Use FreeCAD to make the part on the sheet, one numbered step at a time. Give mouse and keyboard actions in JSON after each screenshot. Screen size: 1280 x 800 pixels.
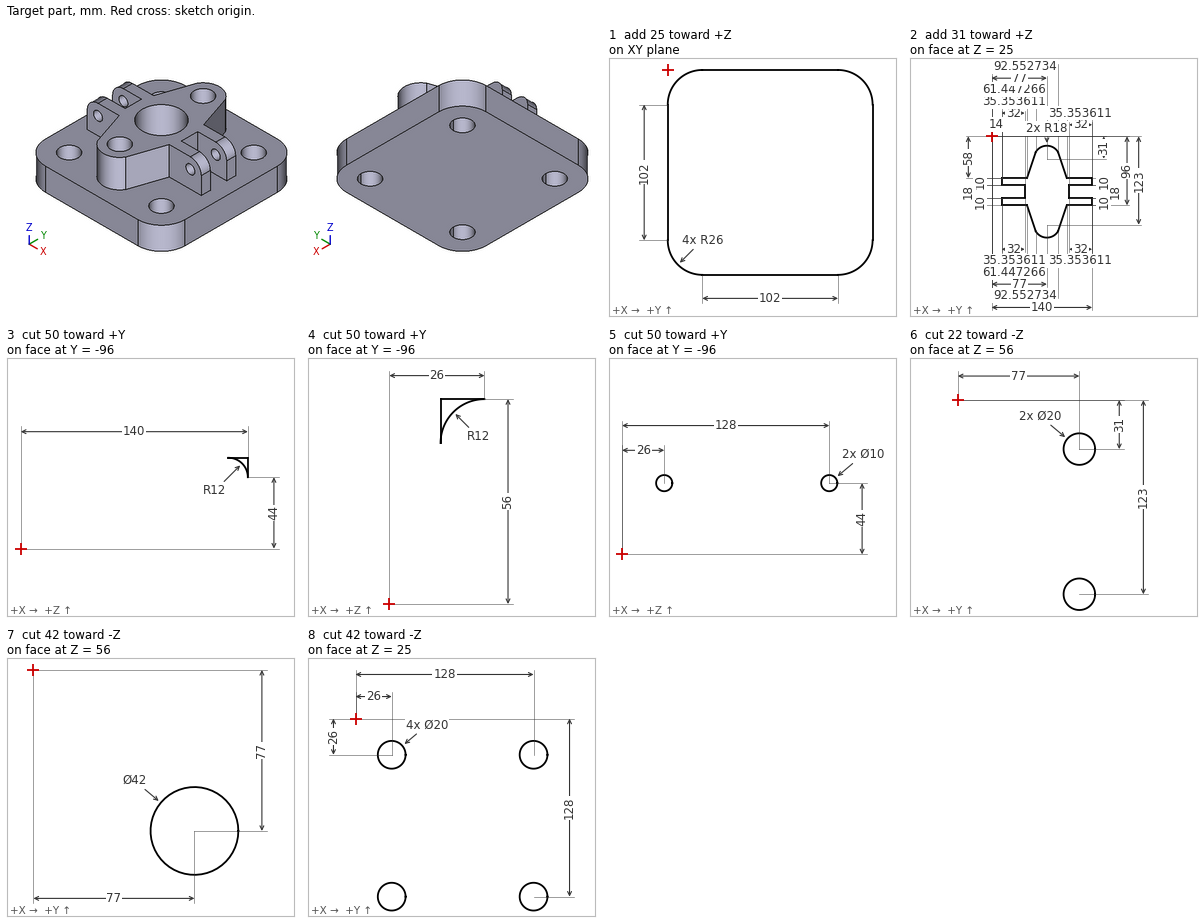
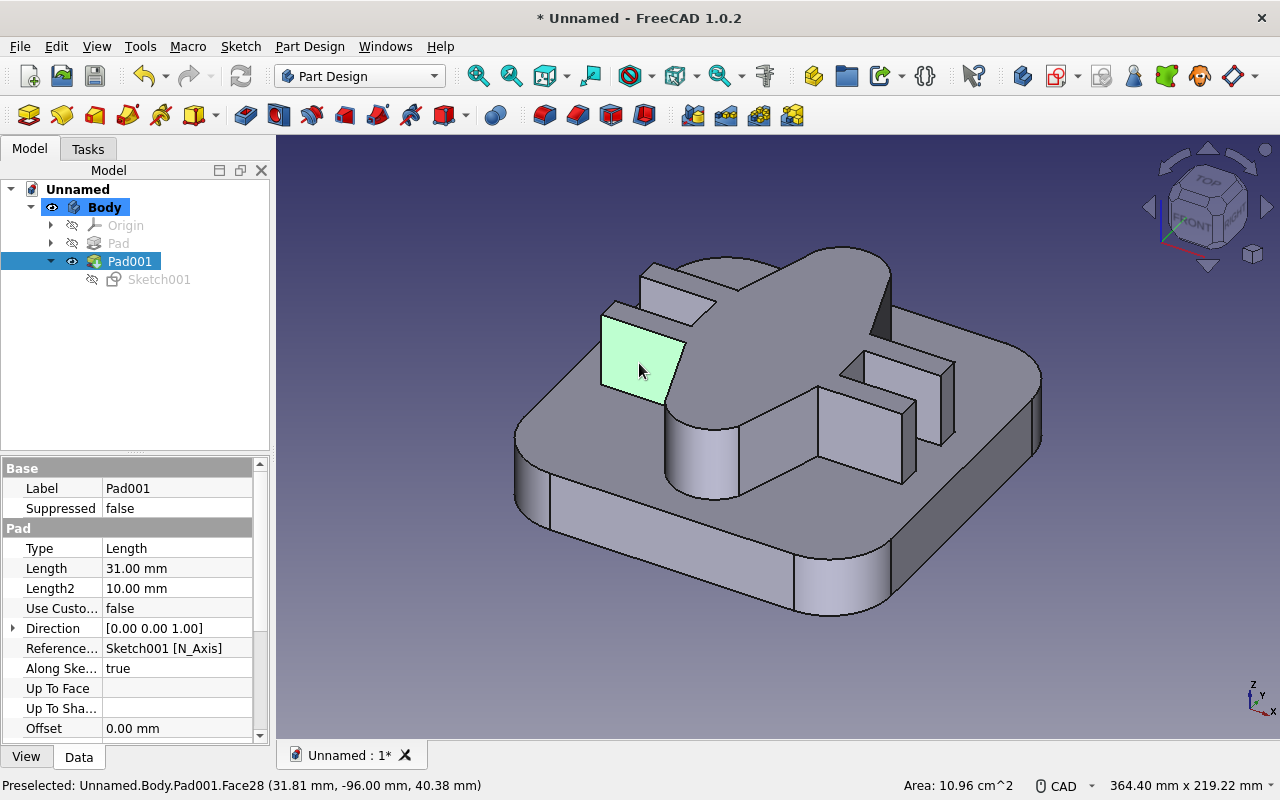
{"action": "left_click", "coordinate": [1056, 76]}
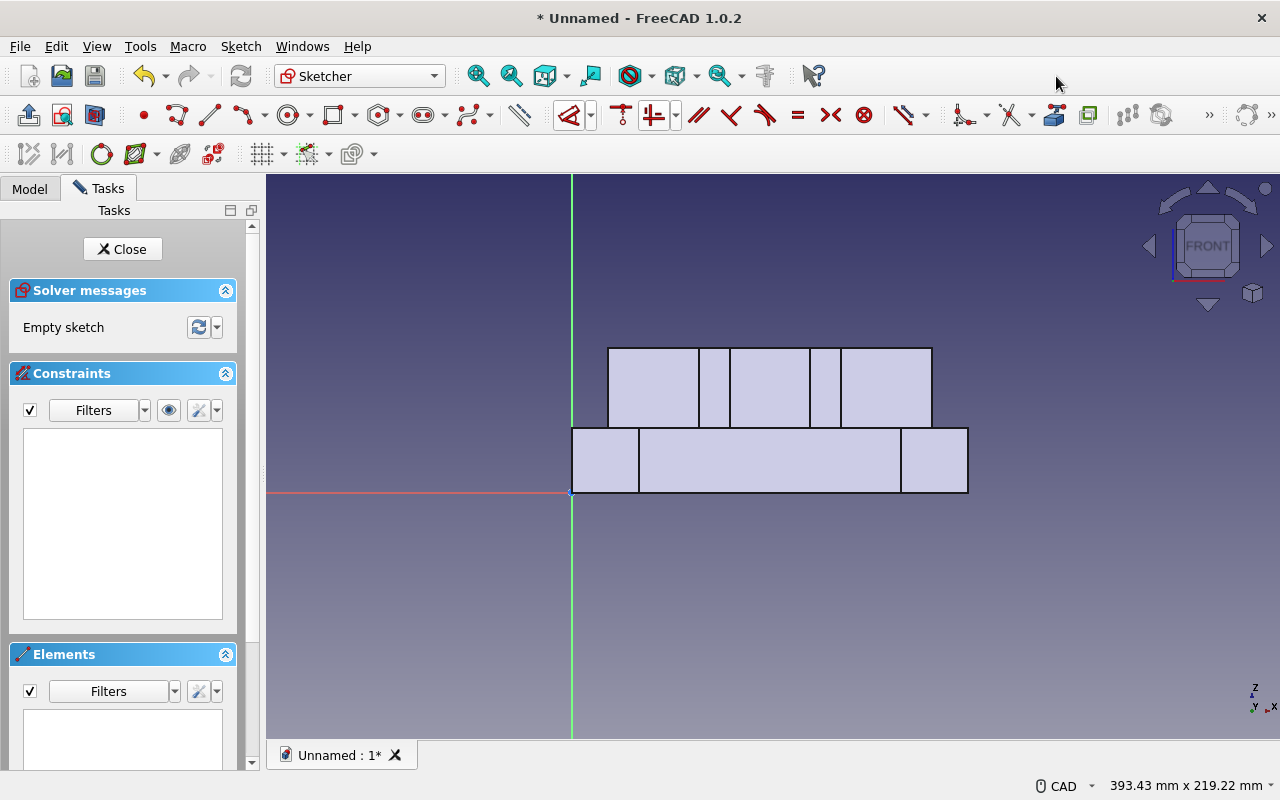
{"action": "scroll", "coordinate": [938, 354], "scroll_direction": "up", "scroll_amount": 12}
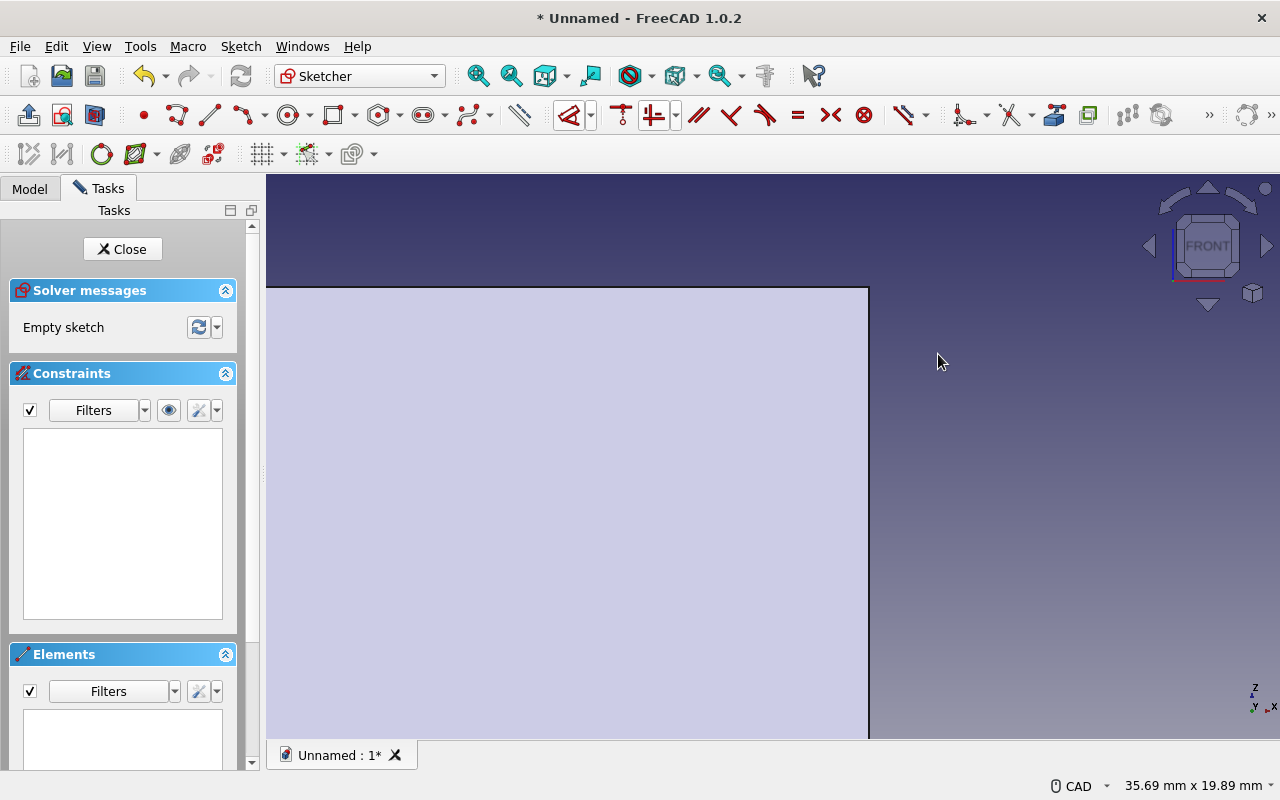
{"action": "left_click", "coordinate": [177, 116]}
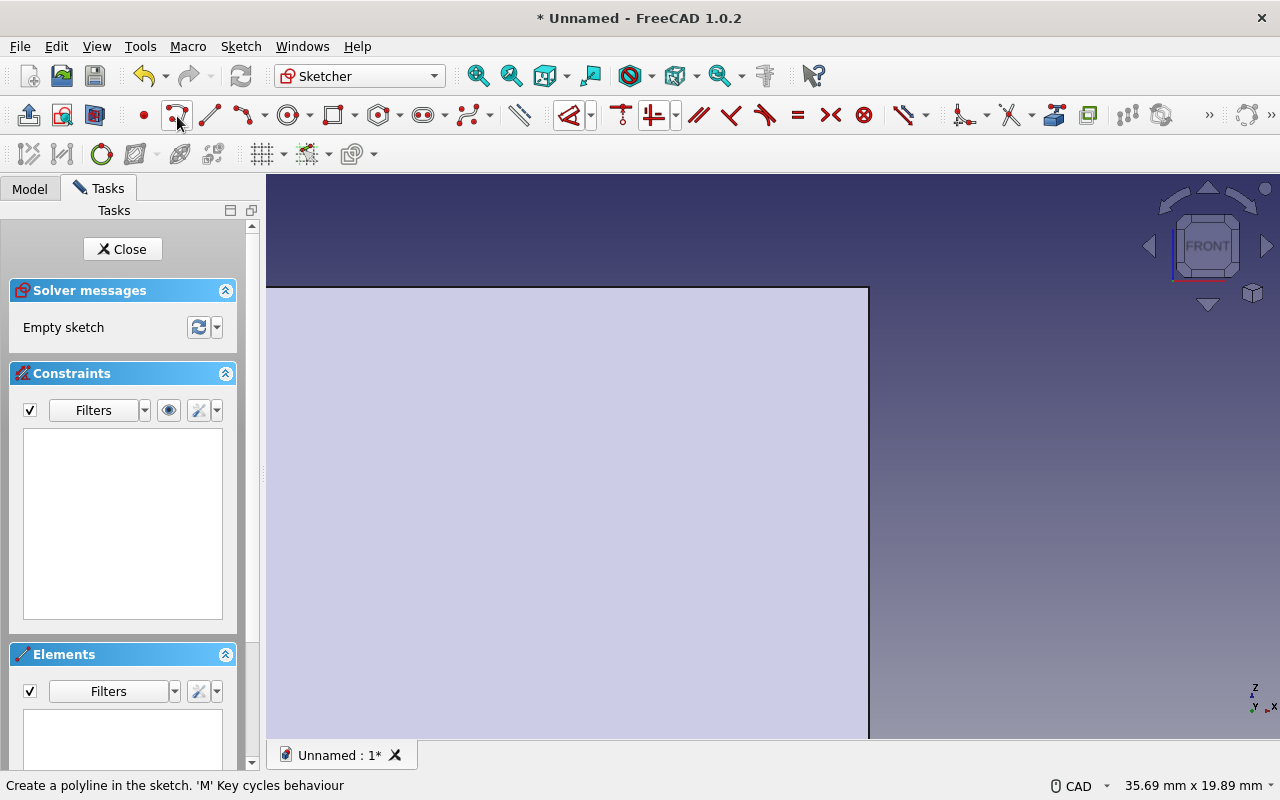
{"action": "left_click", "coordinate": [869, 628]}
{"action": "left_click", "coordinate": [869, 287]}
{"action": "left_click", "coordinate": [528, 287]}
{"action": "right_click", "coordinate": [528, 287]}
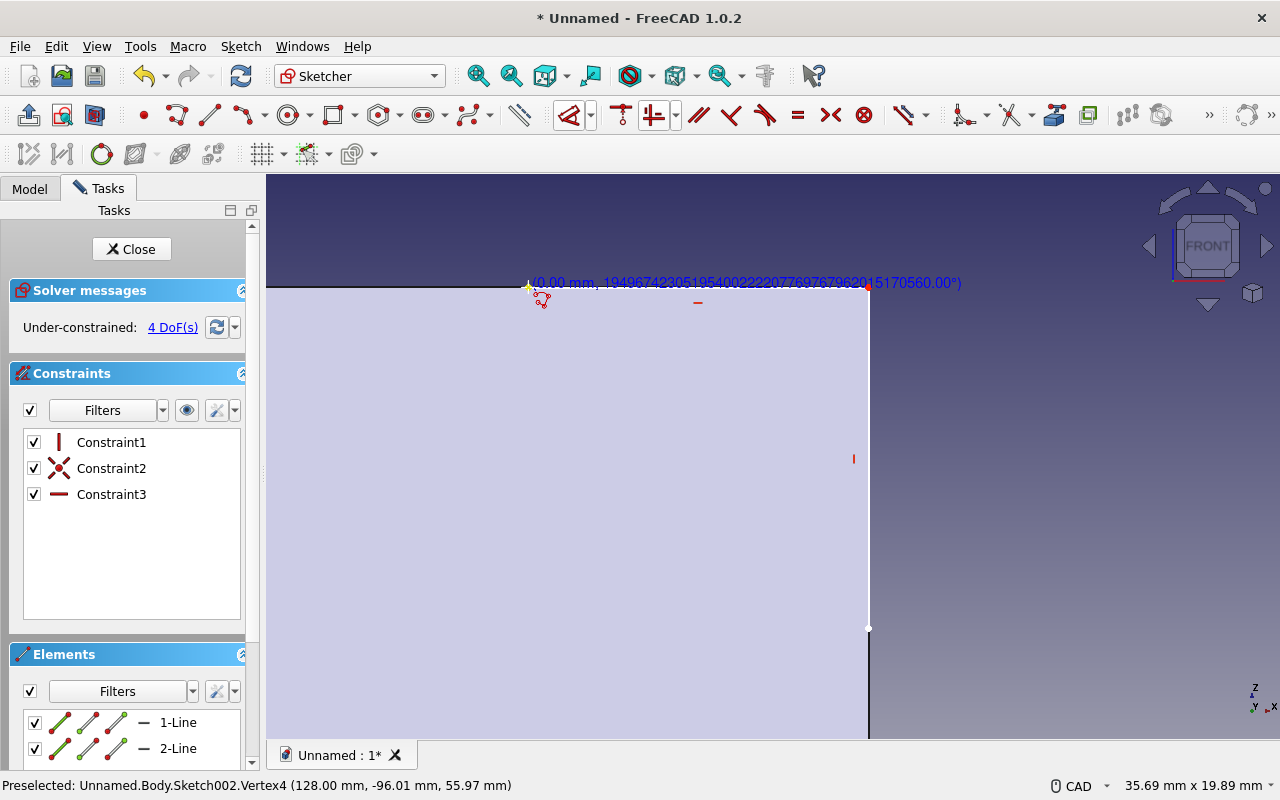
{"action": "left_click", "coordinate": [242, 116]}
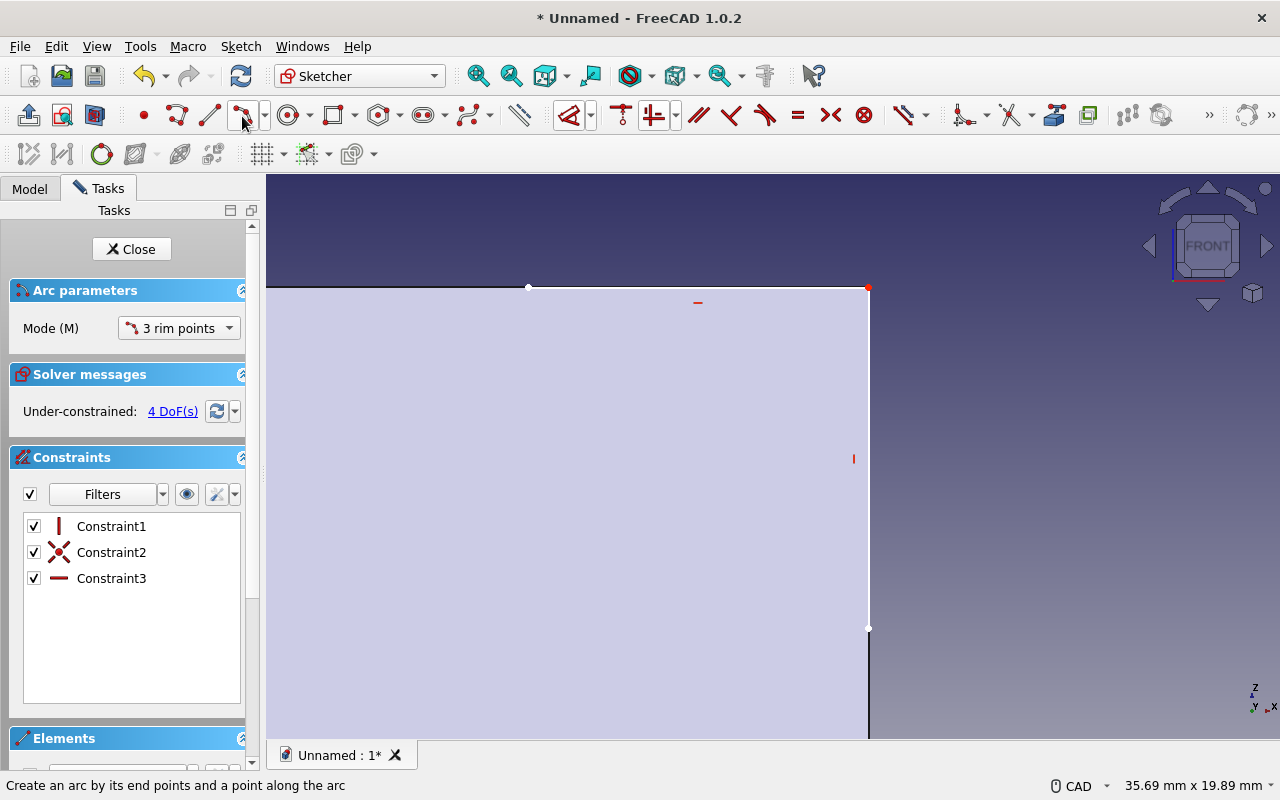
{"action": "left_click", "coordinate": [528, 288]}
{"action": "left_click", "coordinate": [869, 629]}
{"action": "left_click", "coordinate": [769, 387]}
{"action": "key", "text": "Escape"}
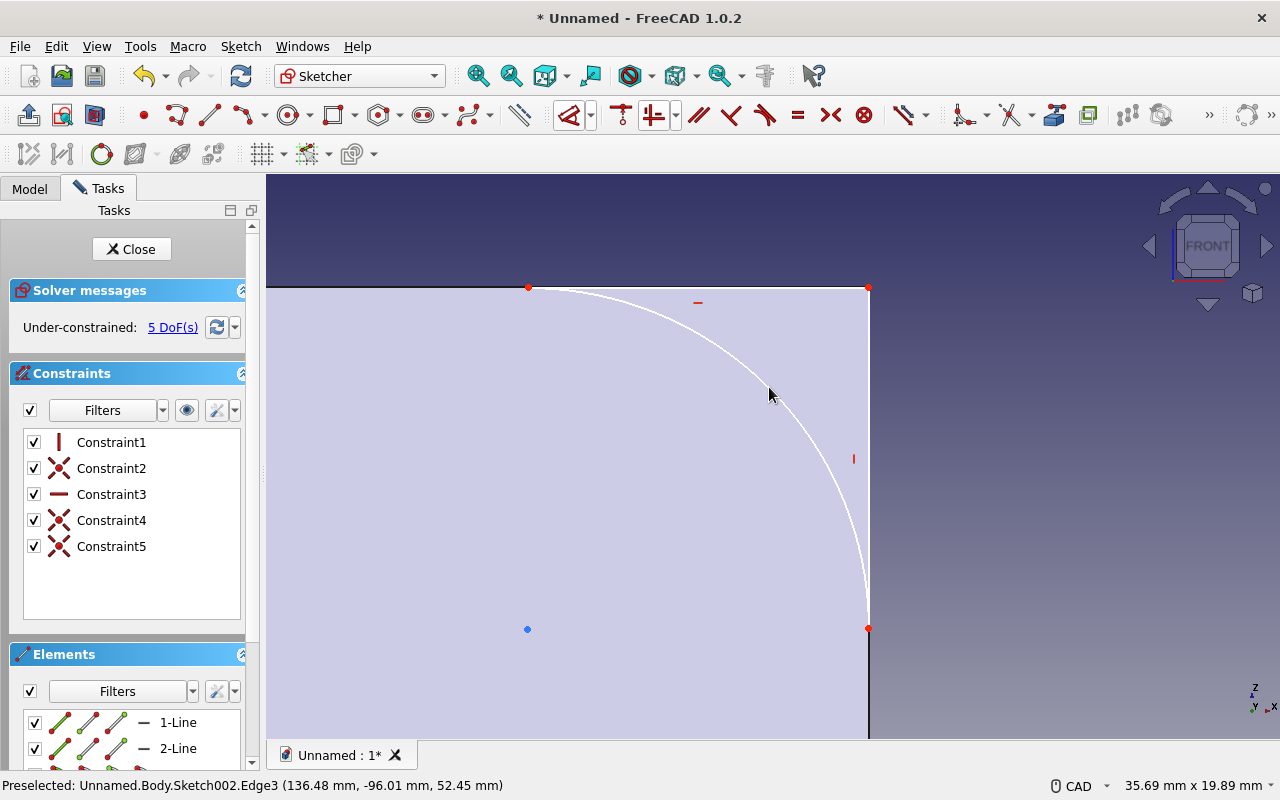
{"action": "left_click", "coordinate": [869, 527]}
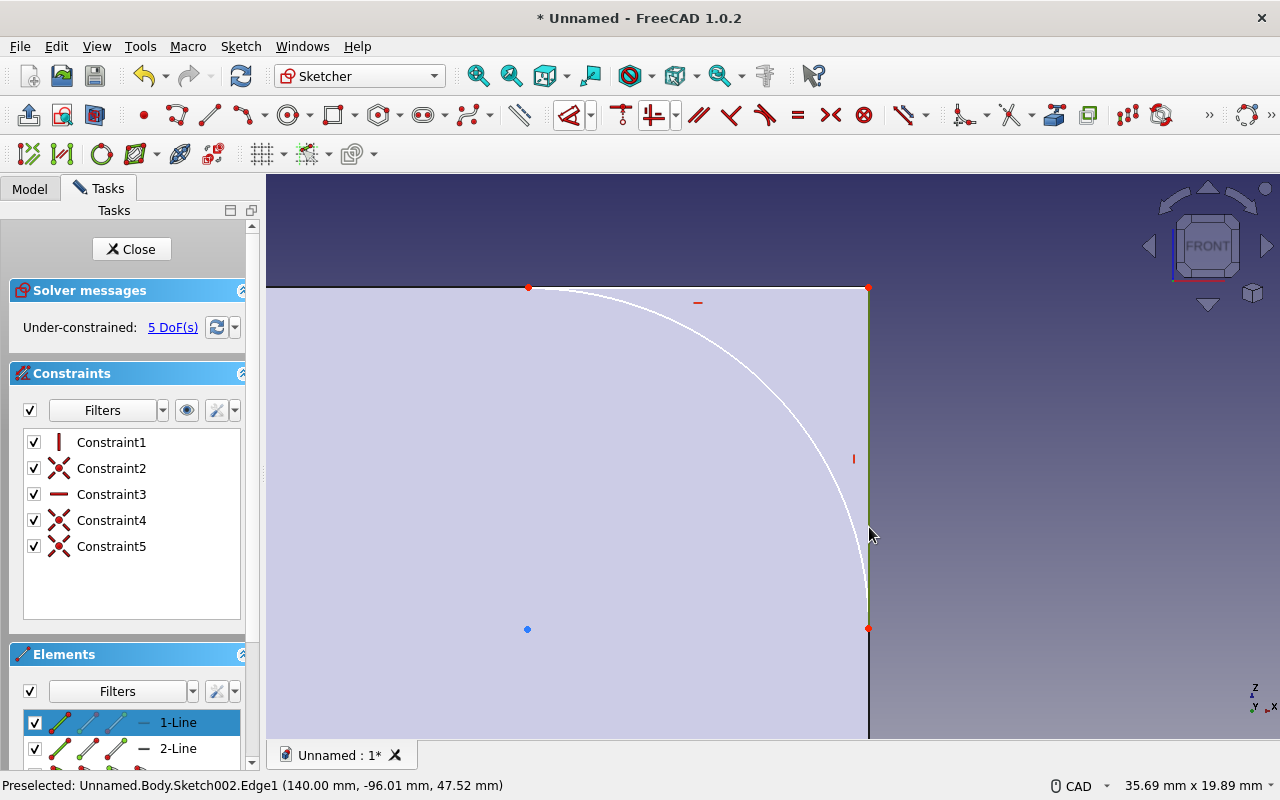
{"action": "left_click", "coordinate": [832, 474]}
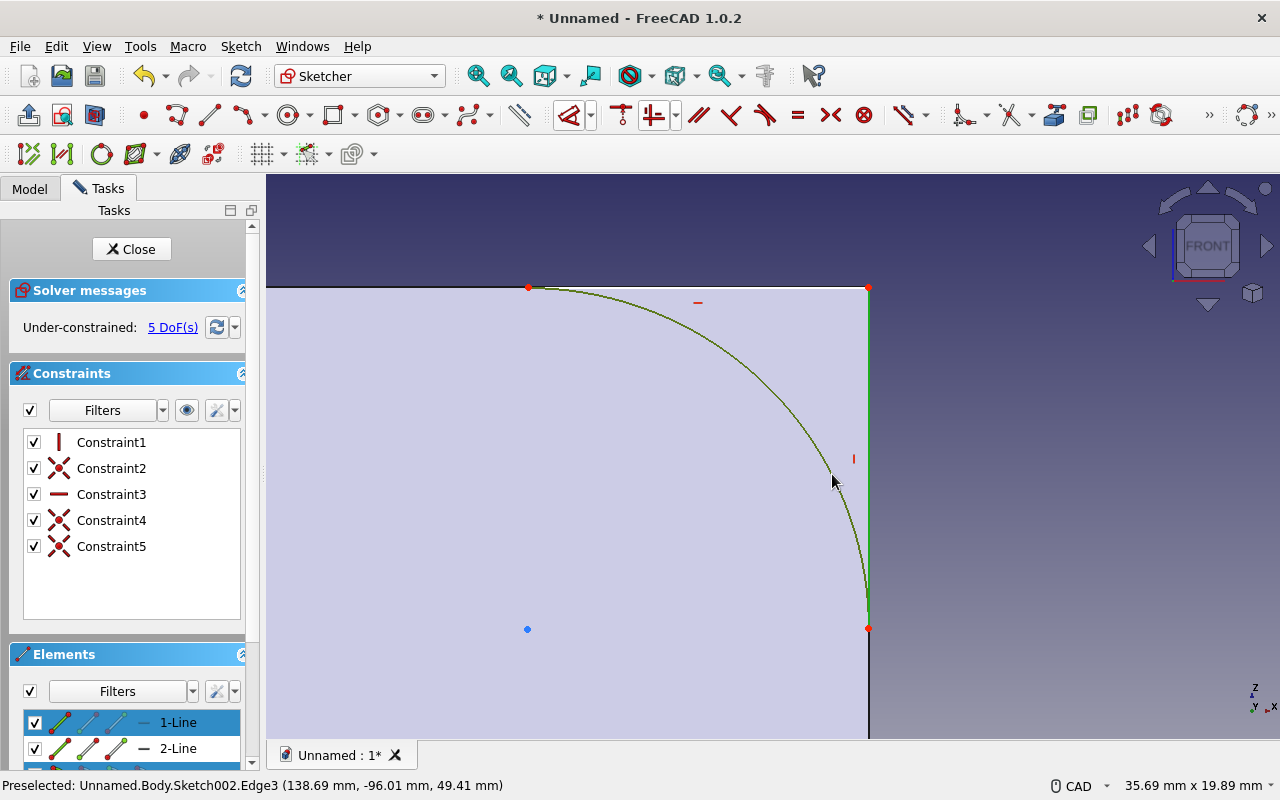
{"action": "left_click", "coordinate": [765, 116]}